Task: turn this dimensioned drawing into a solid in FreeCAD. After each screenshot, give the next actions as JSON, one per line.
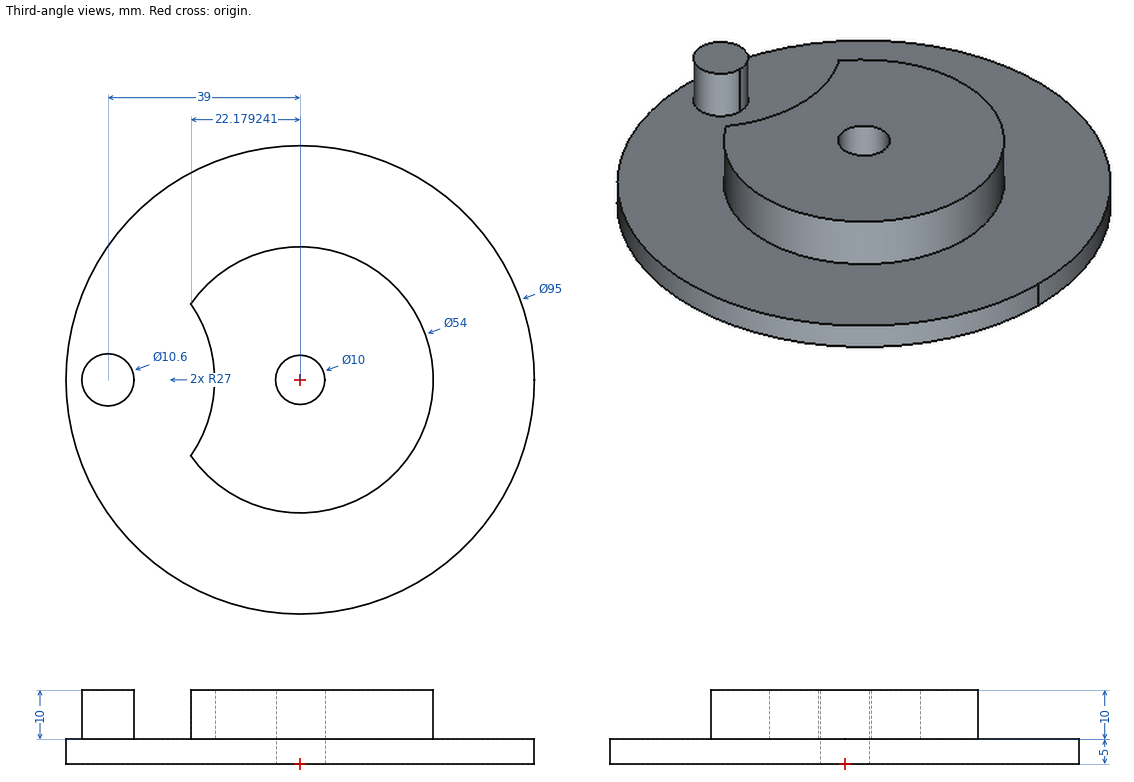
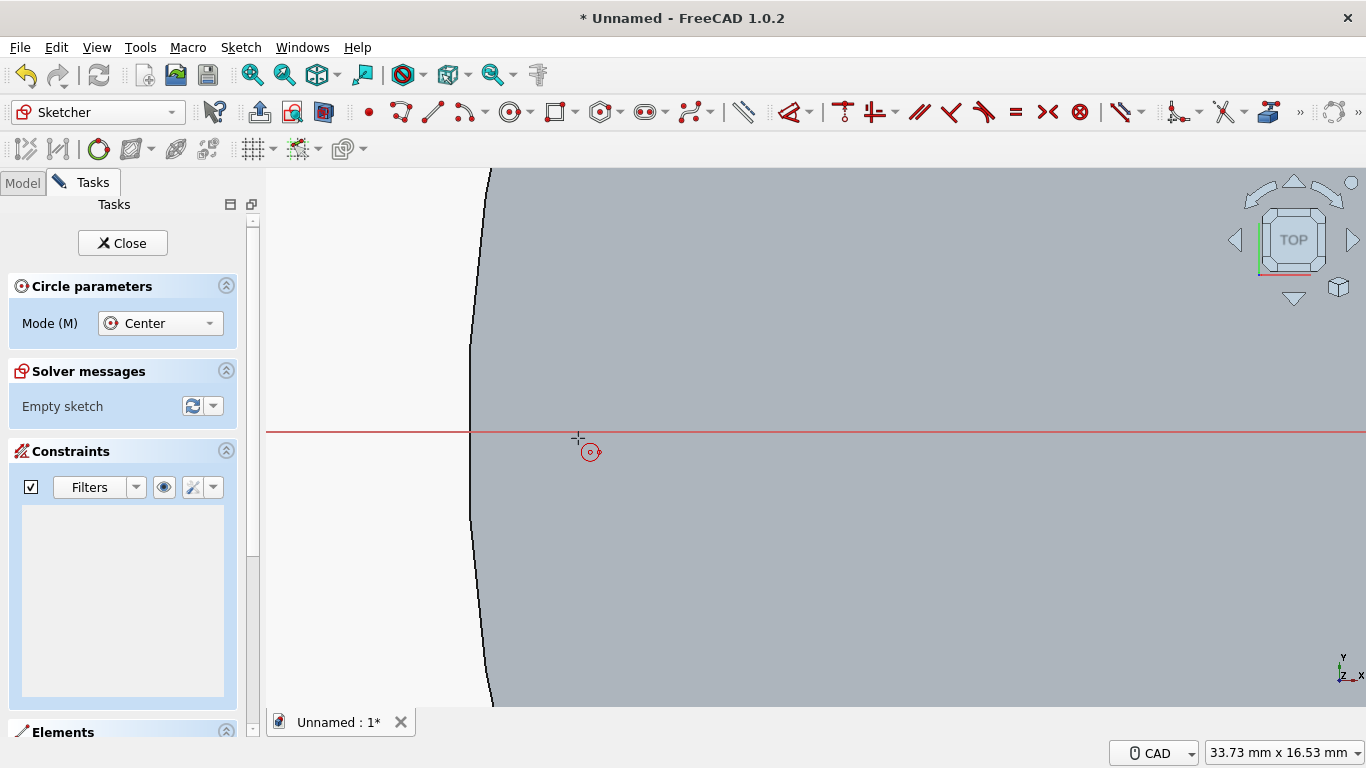
{"action": "left_click", "coordinate": [745, 432]}
{"action": "left_click", "coordinate": [867, 310]}
{"action": "key", "text": "Escape"}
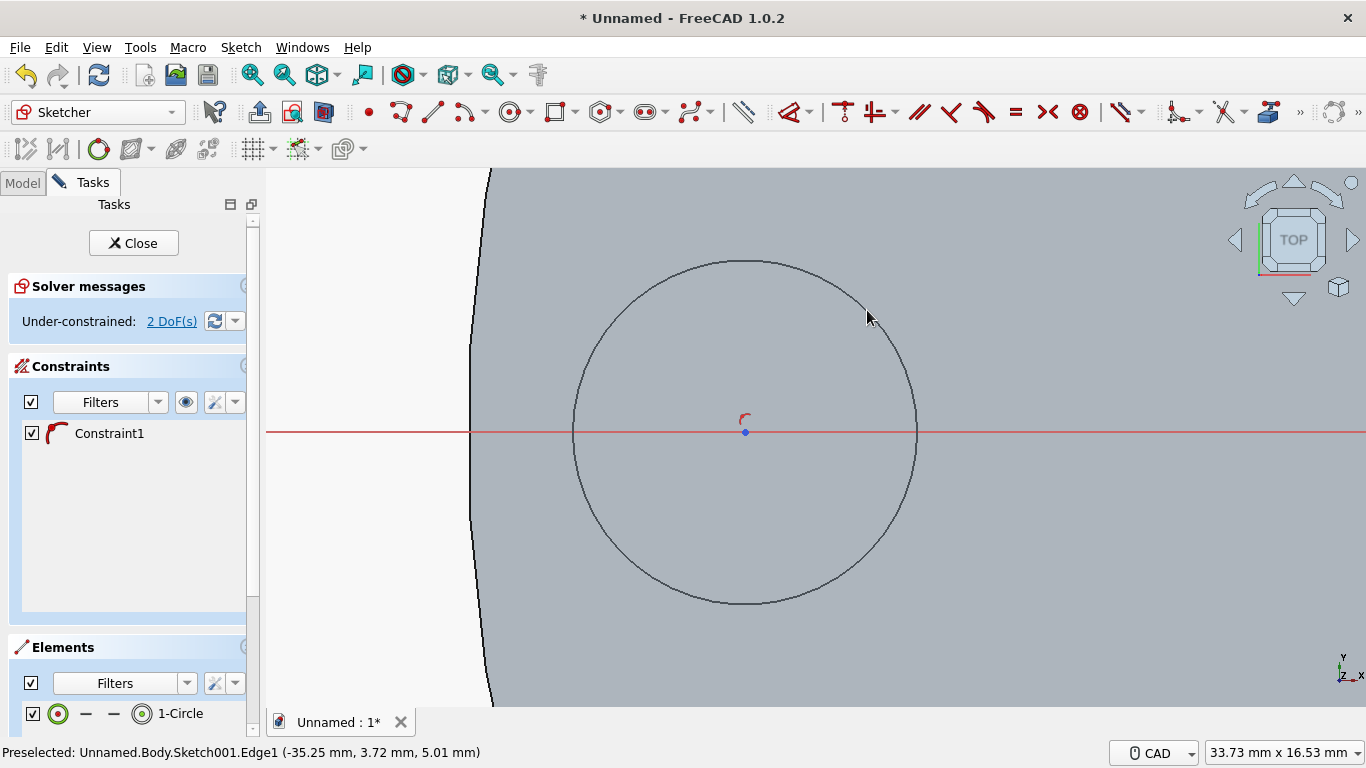
{"action": "key", "text": "d"}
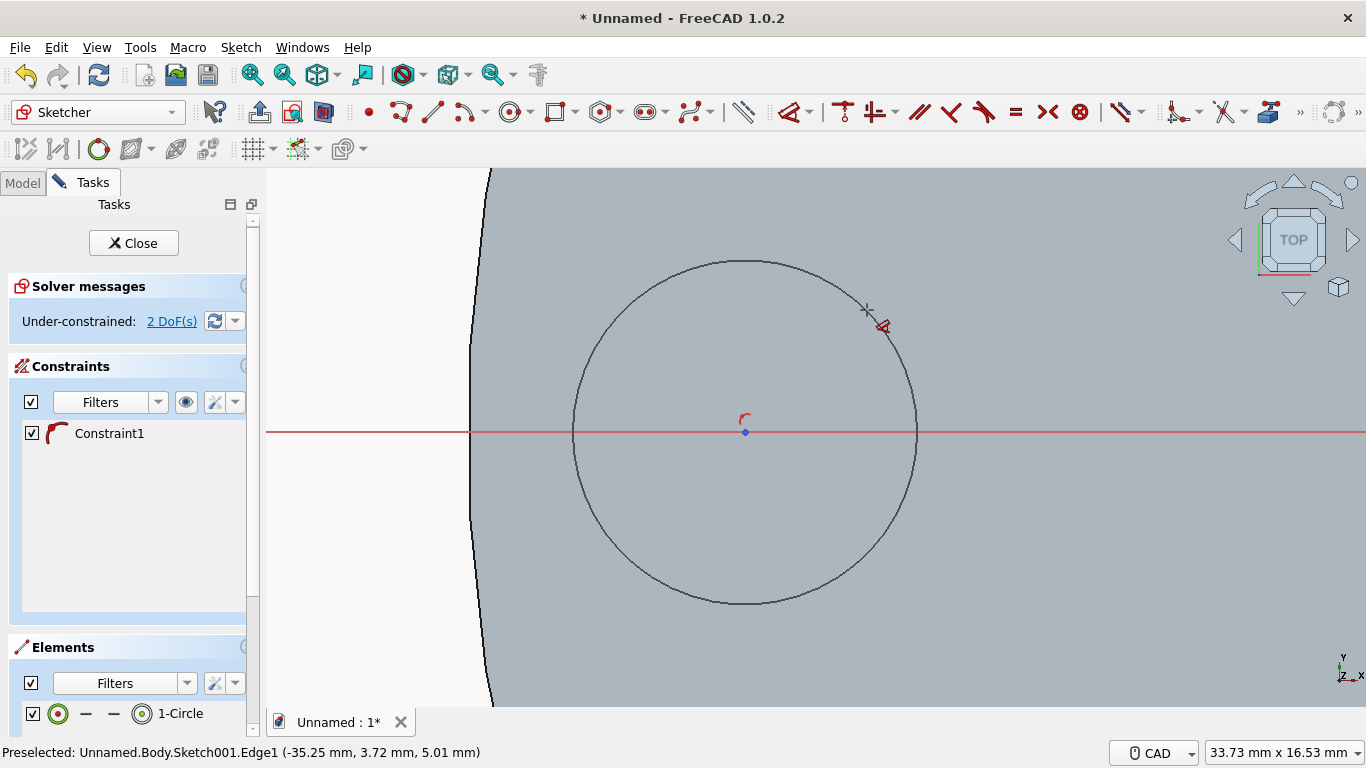
{"action": "left_click", "coordinate": [866, 310]}
{"action": "left_click", "coordinate": [888, 287]}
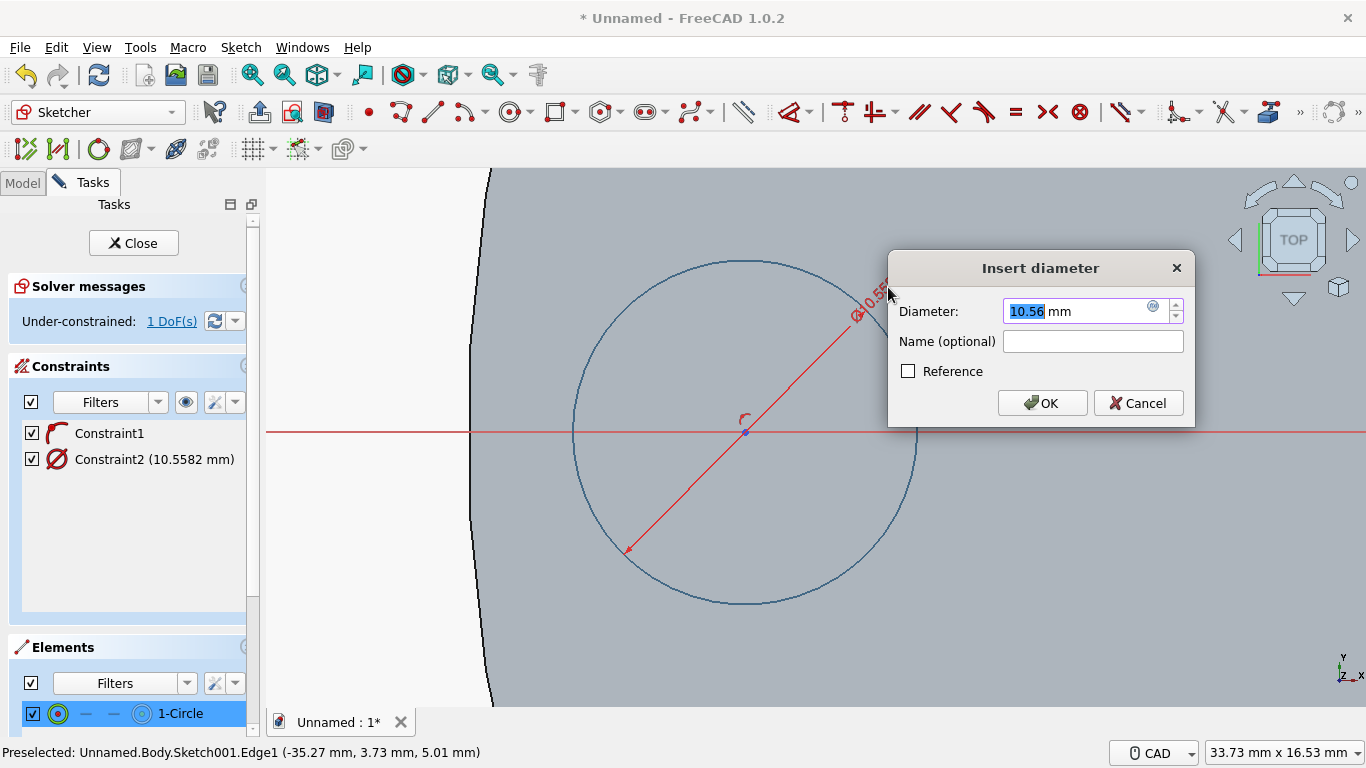
{"action": "type", "text": "10.6"}
{"action": "key", "text": "Return"}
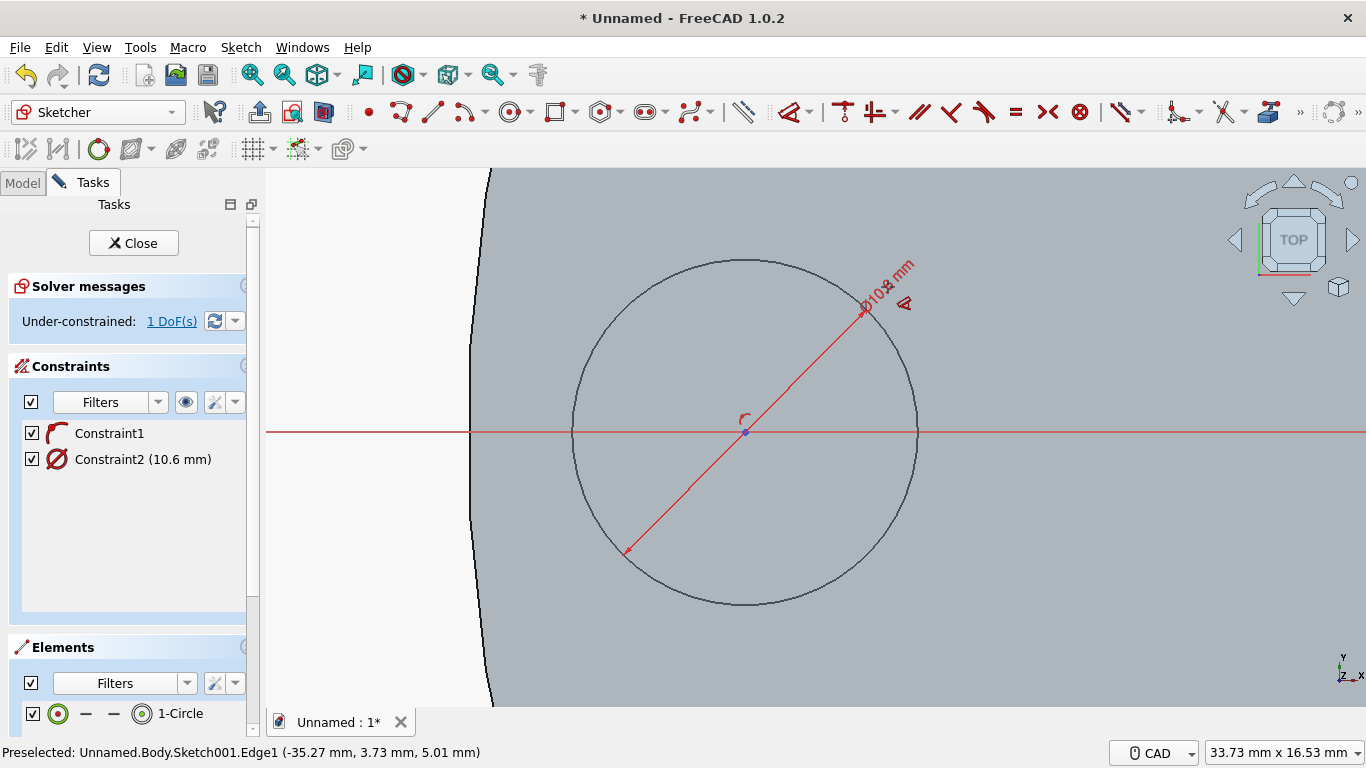
{"action": "left_click", "coordinate": [745, 432]}
{"action": "left_click", "coordinate": [973, 466]}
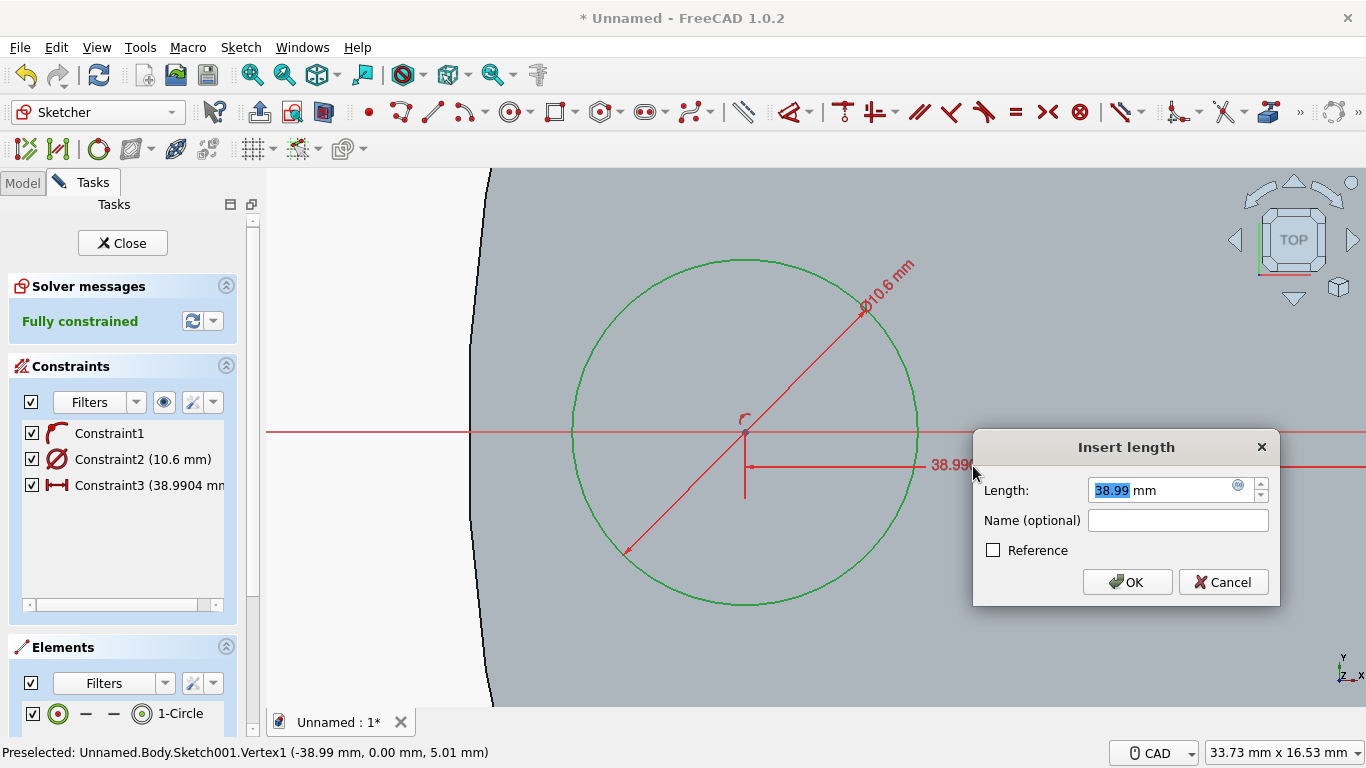
{"action": "type", "text": "39"}
{"action": "key", "text": "Return"}
{"action": "key", "text": "Escape"}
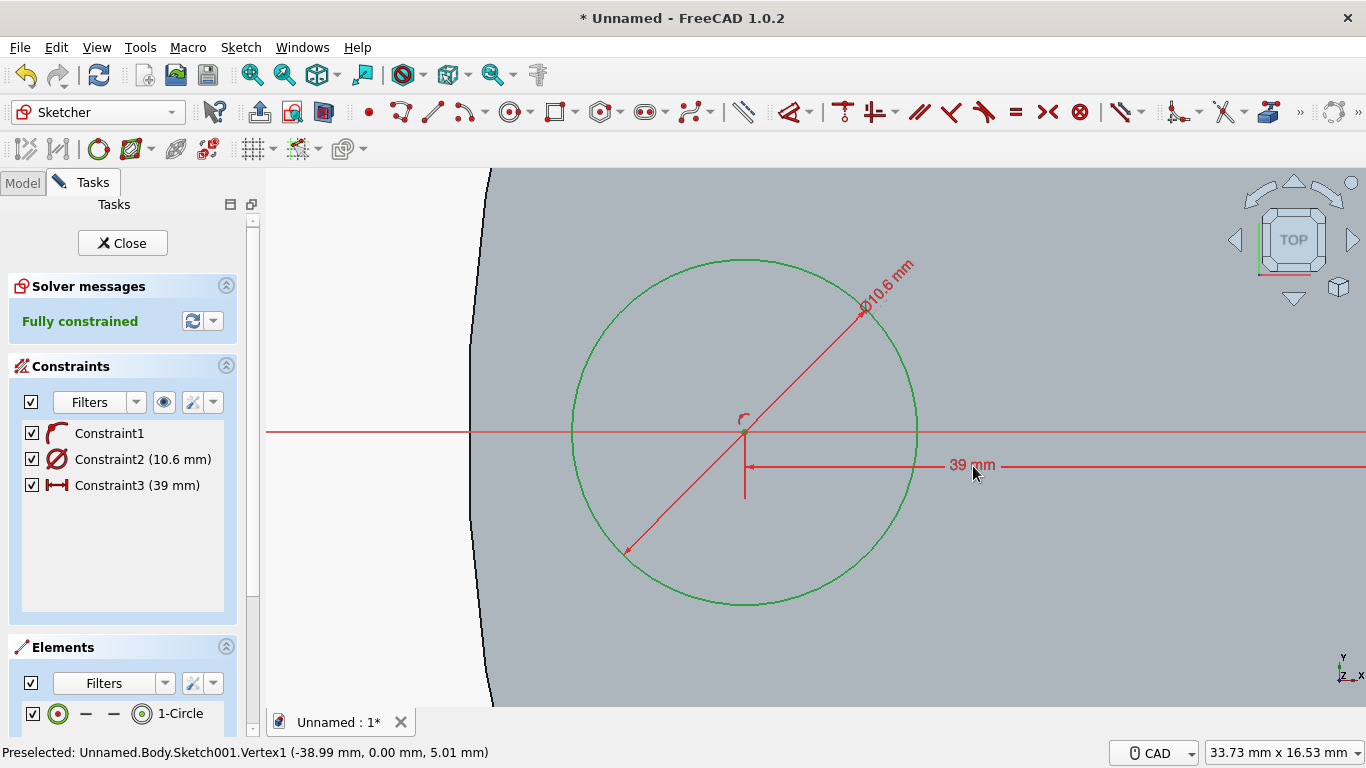
{"action": "left_click", "coordinate": [123, 243]}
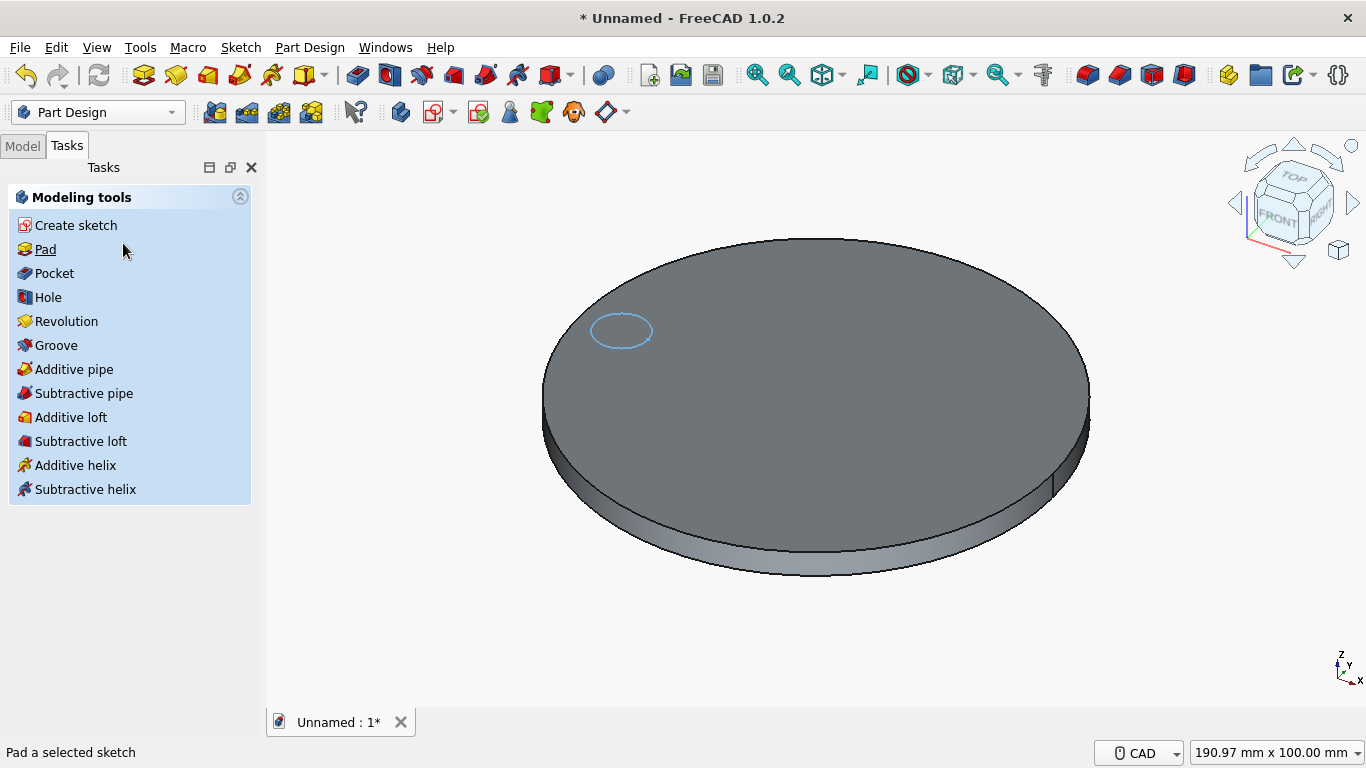
{"action": "left_click", "coordinate": [144, 76]}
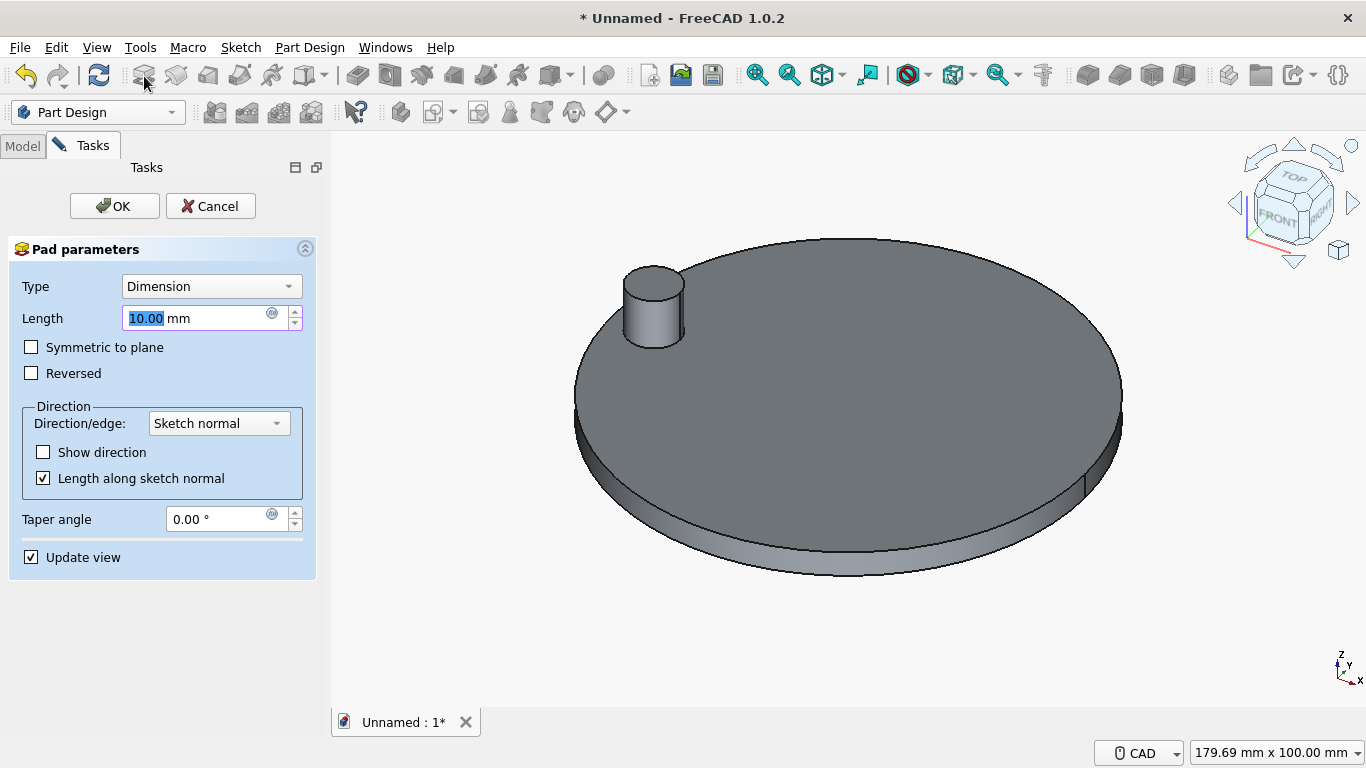
{"action": "type", "text": "10"}
{"action": "key", "text": "Tab"}